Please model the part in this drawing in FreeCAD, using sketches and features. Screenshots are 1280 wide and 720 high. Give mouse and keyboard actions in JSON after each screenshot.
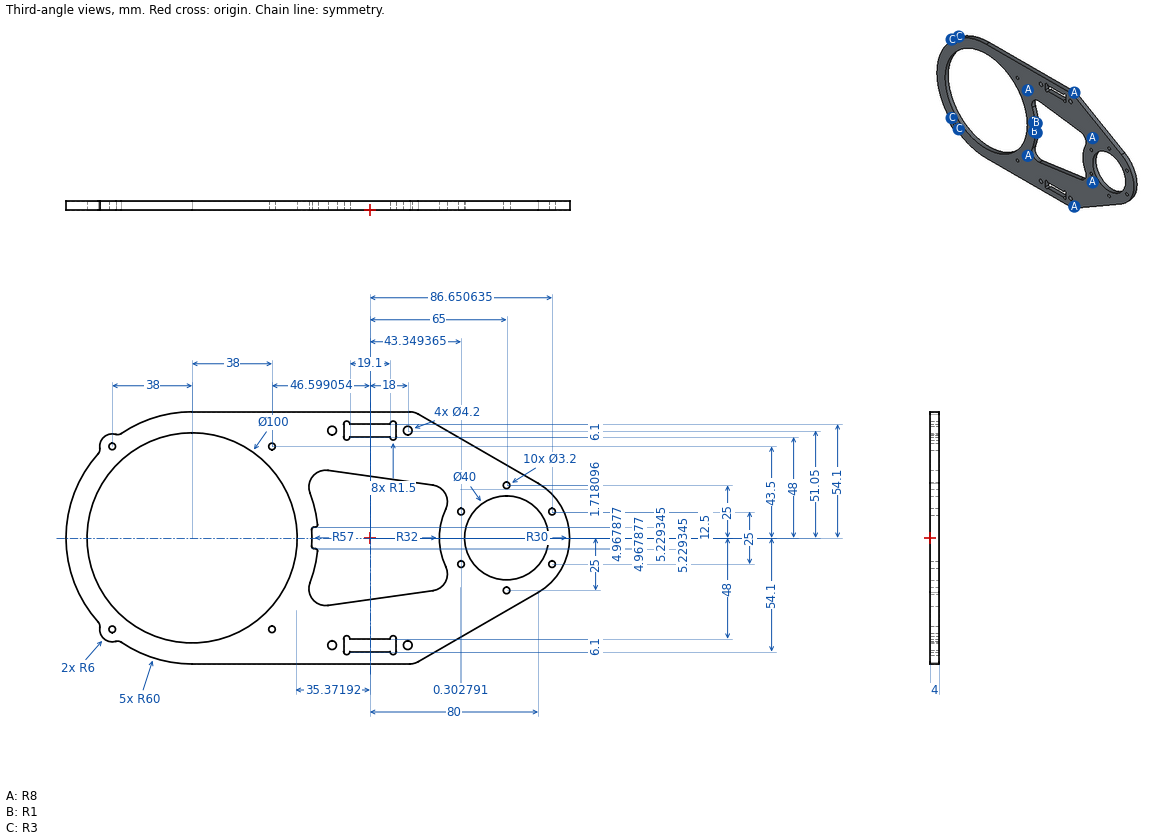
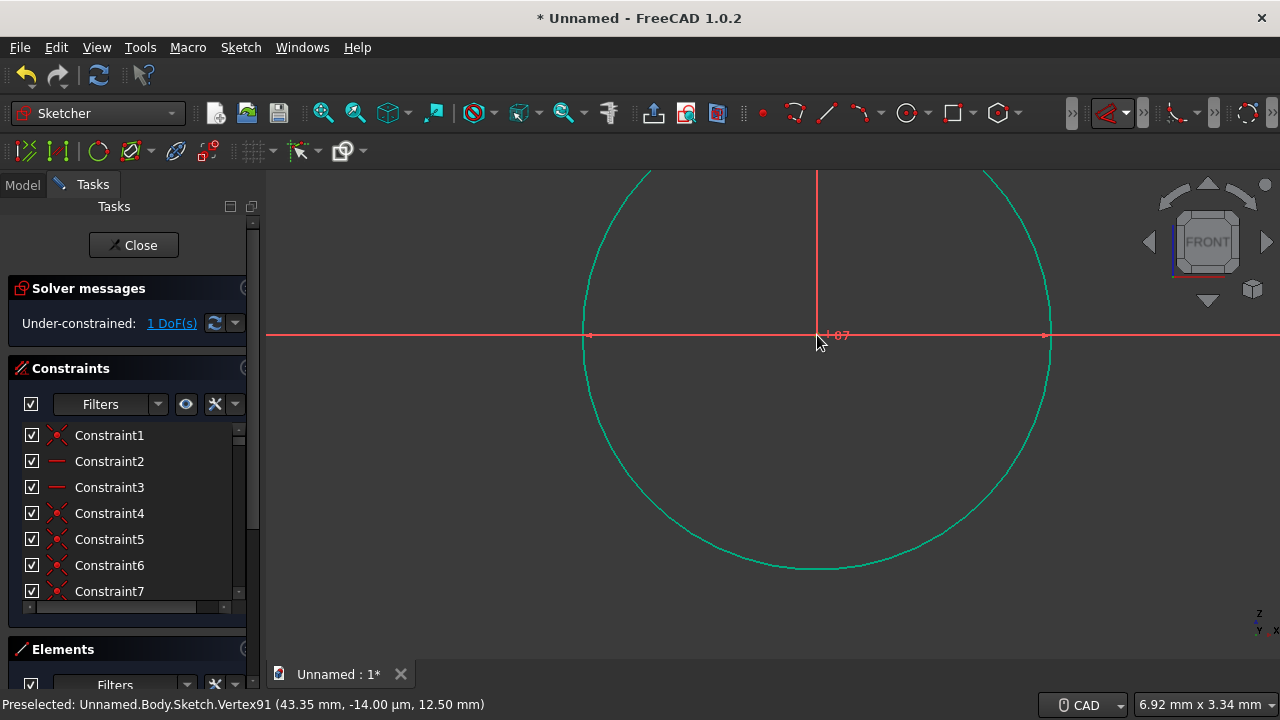
{"action": "left_click", "coordinate": [1128, 114]}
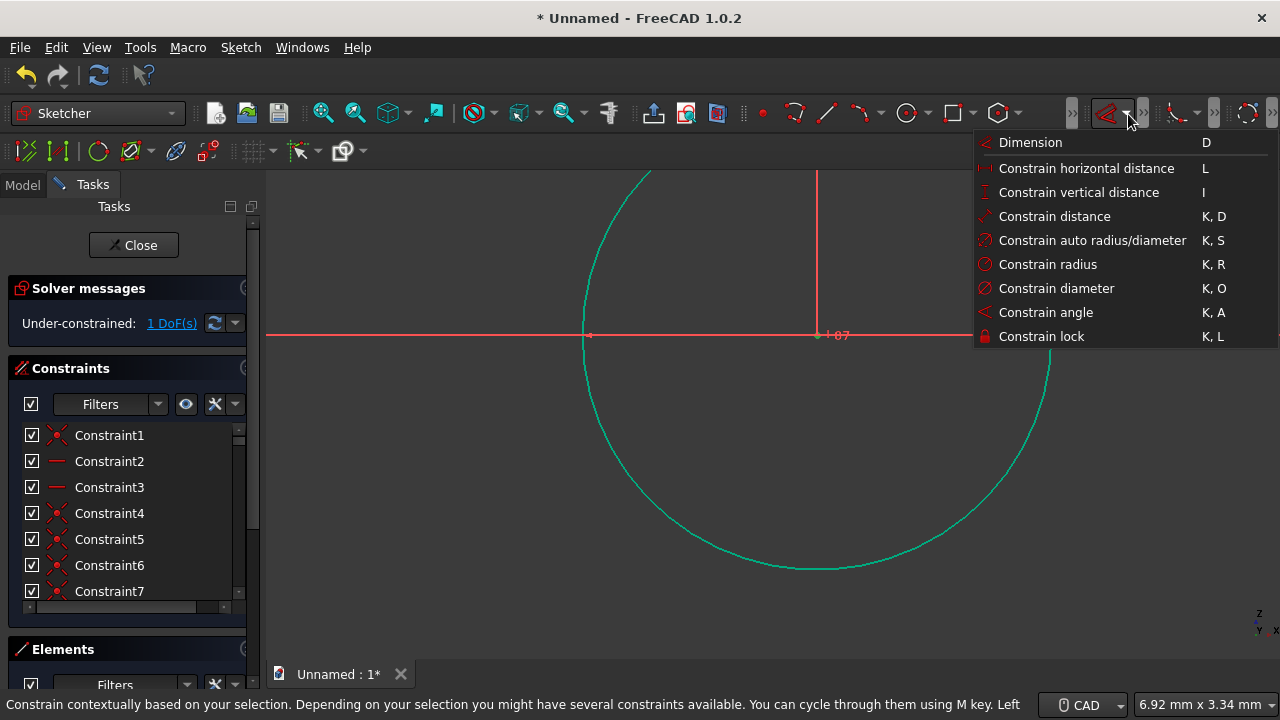
{"action": "left_click", "coordinate": [1126, 168]}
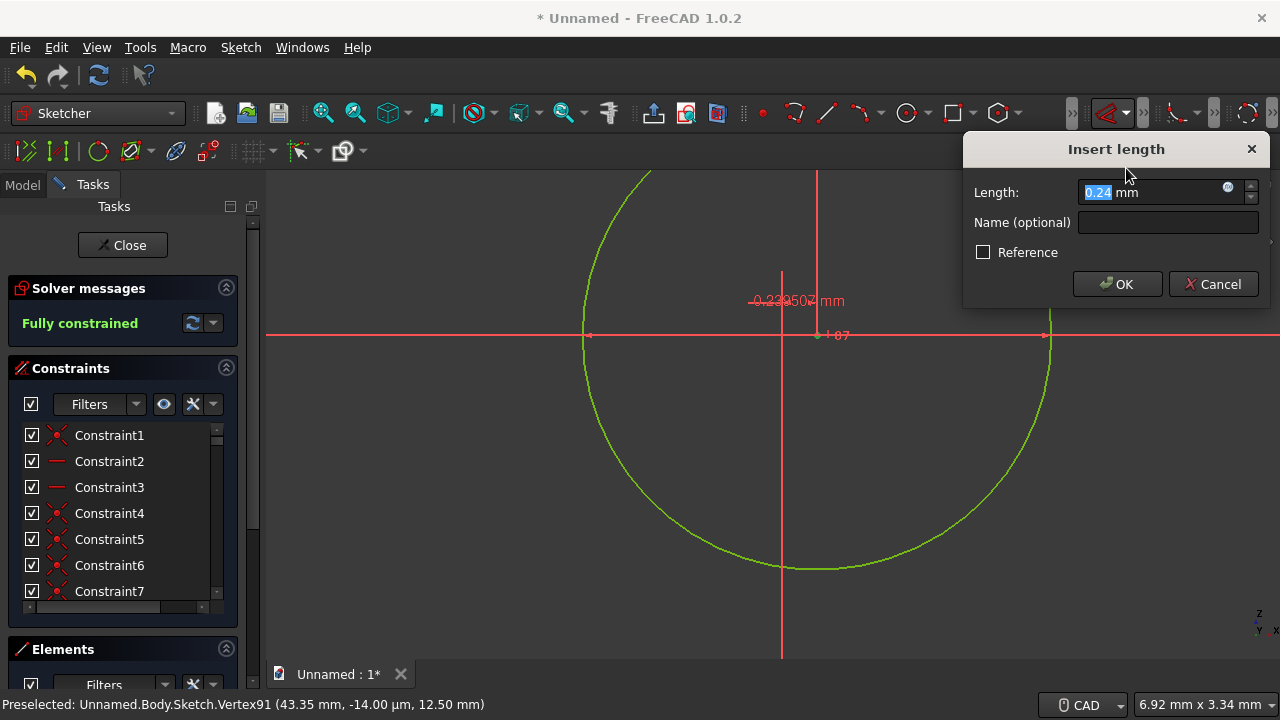
{"action": "type", "text": "0.302791"}
{"action": "key", "text": "Return"}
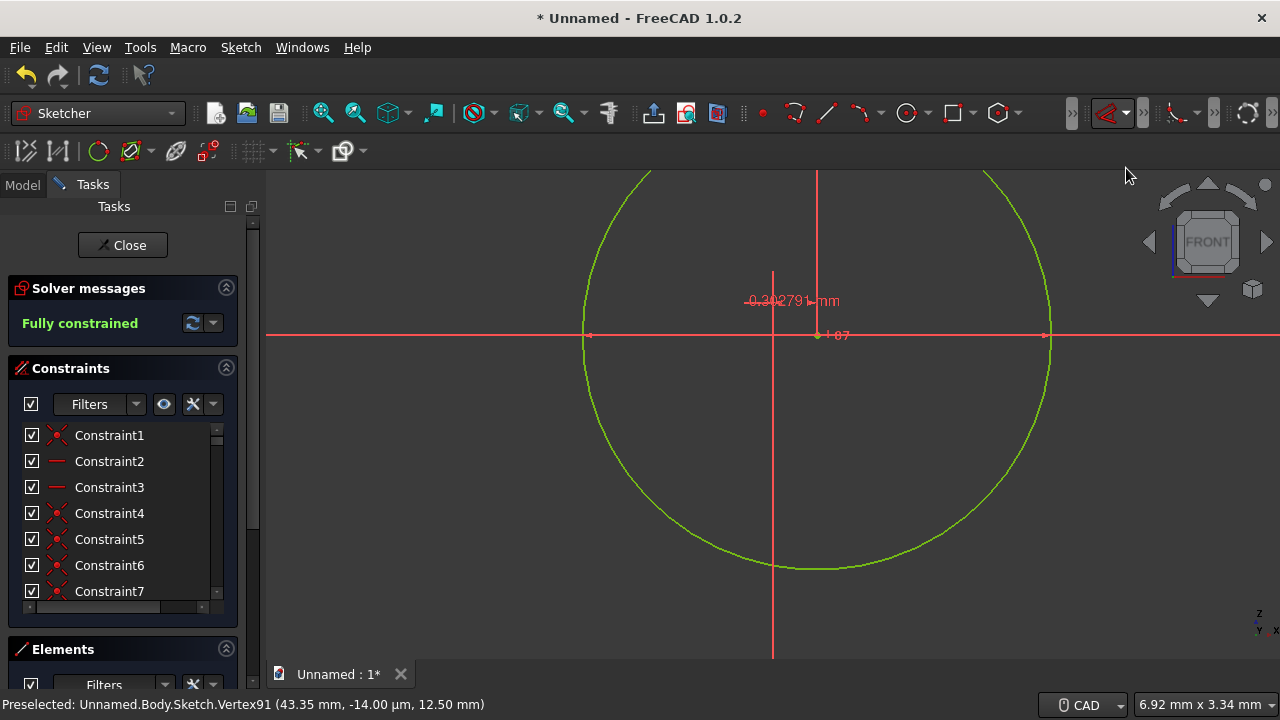
{"action": "left_click", "coordinate": [123, 245]}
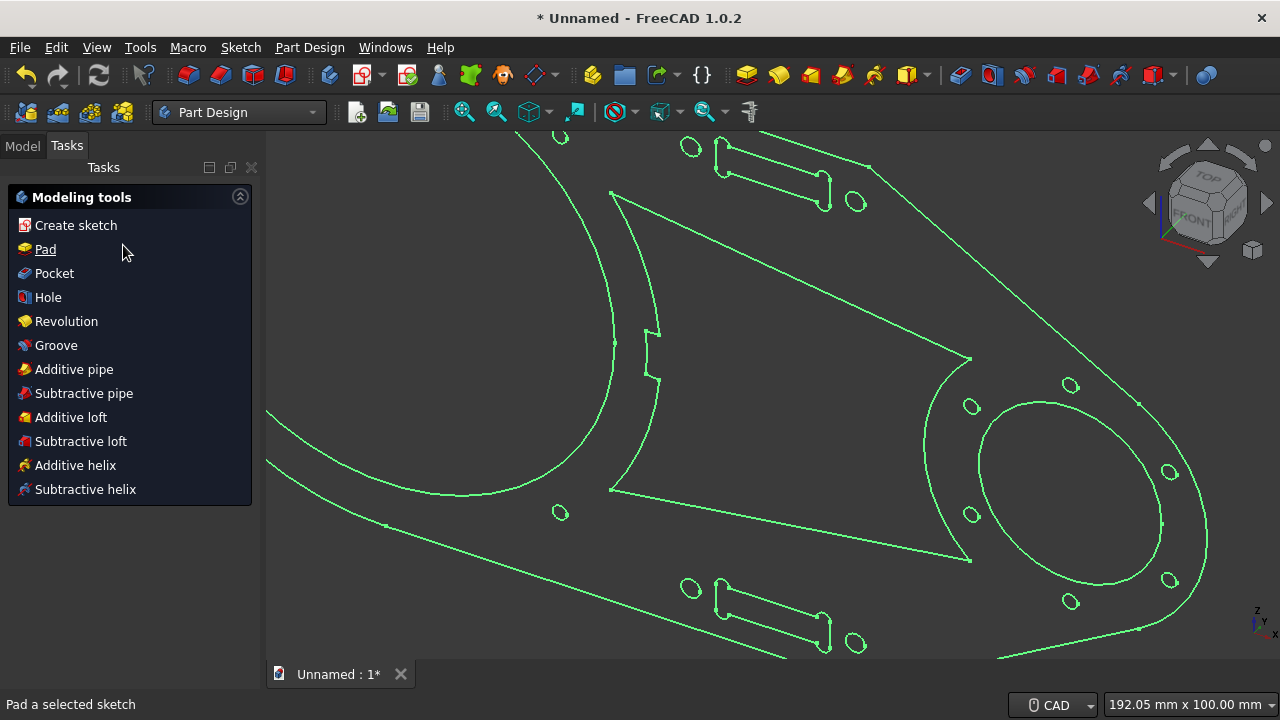
{"action": "left_click", "coordinate": [748, 76]}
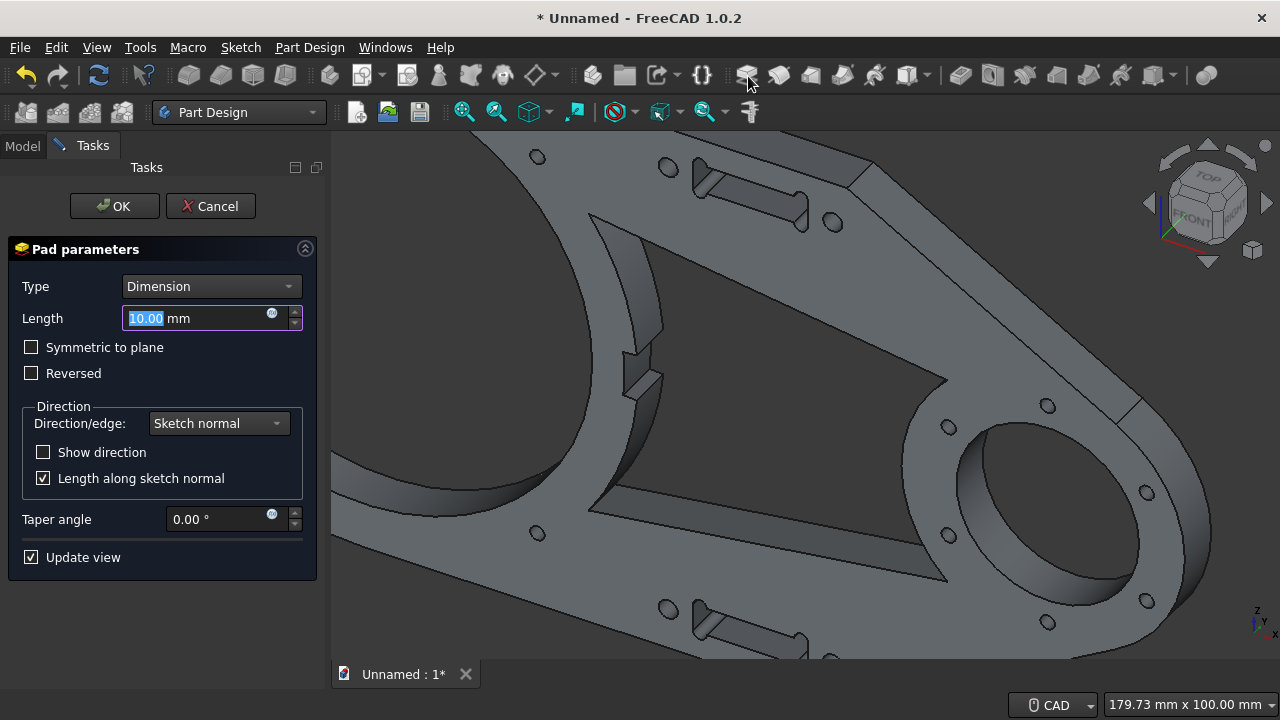
{"action": "type", "text": "4"}
{"action": "key", "text": "Tab"}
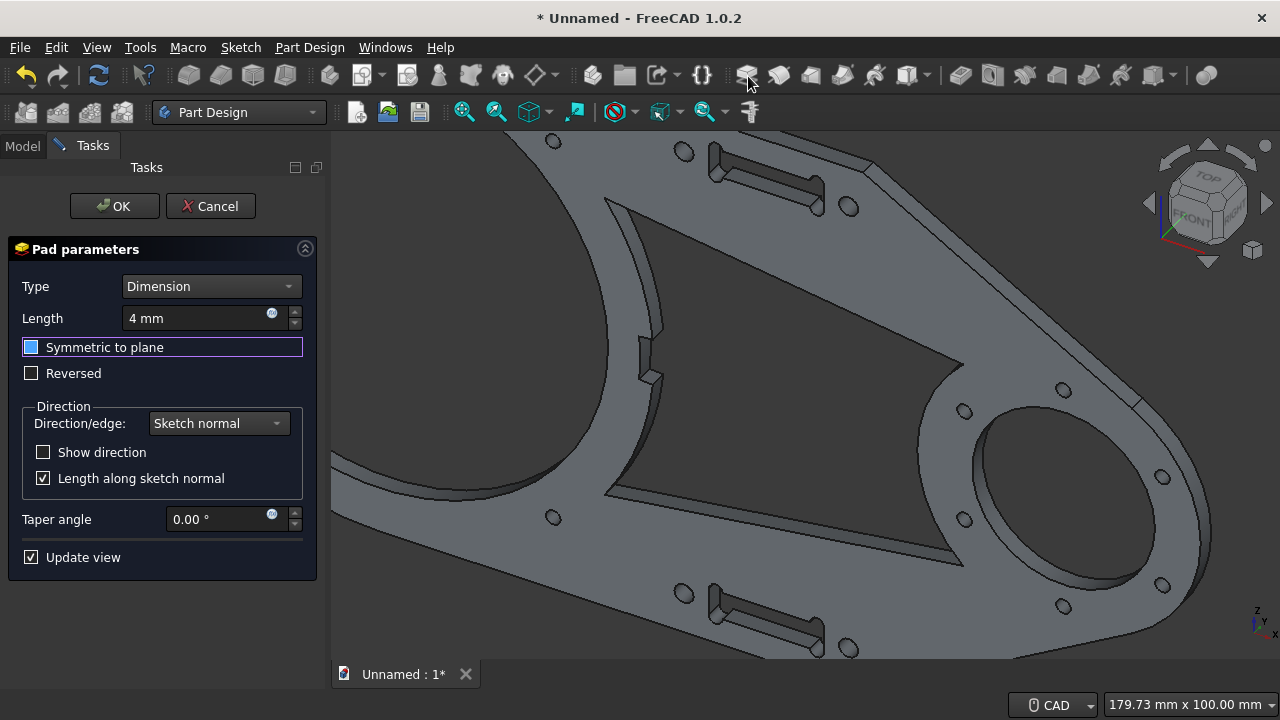
{"action": "left_click", "coordinate": [30, 373]}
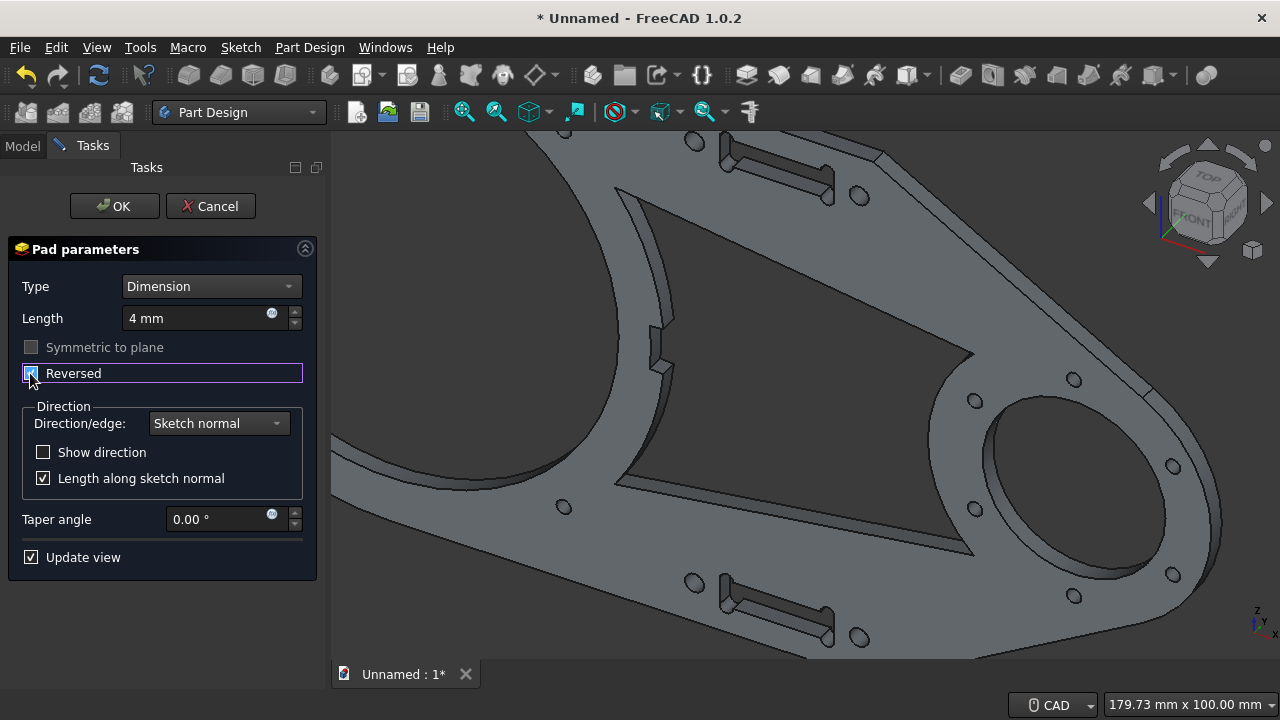
{"action": "left_click", "coordinate": [115, 206]}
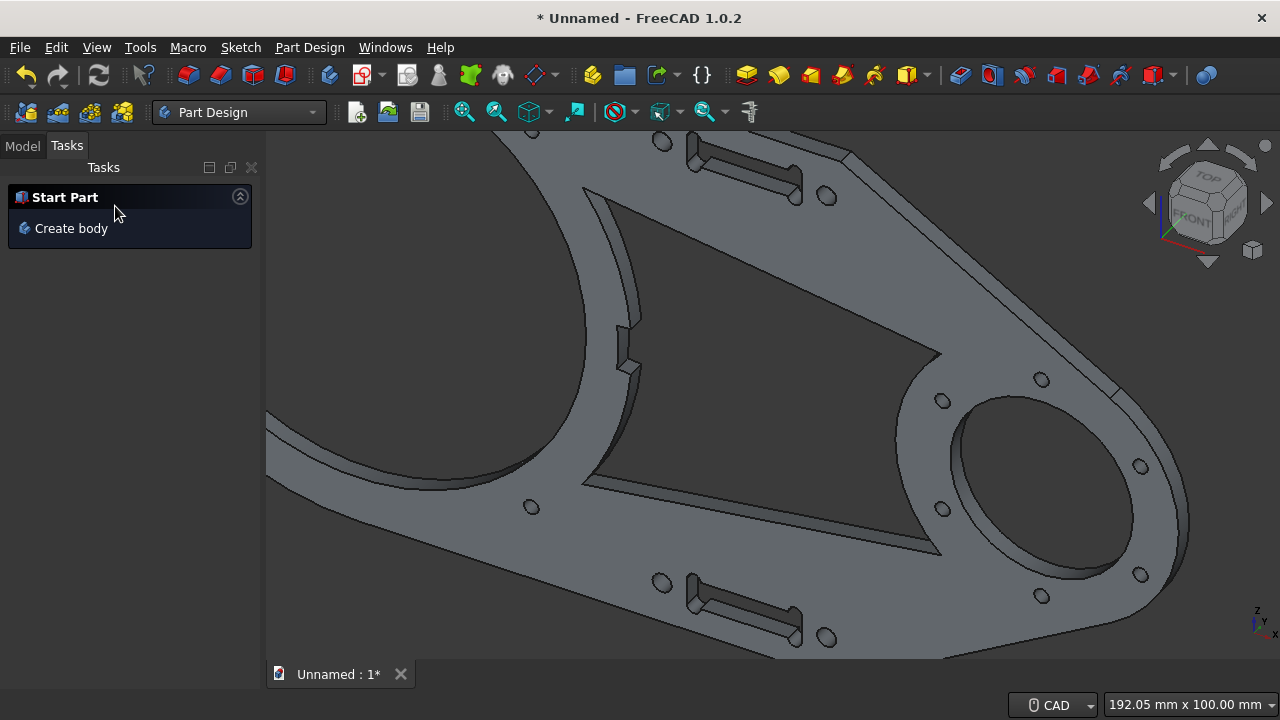
{"action": "left_click", "coordinate": [466, 112]}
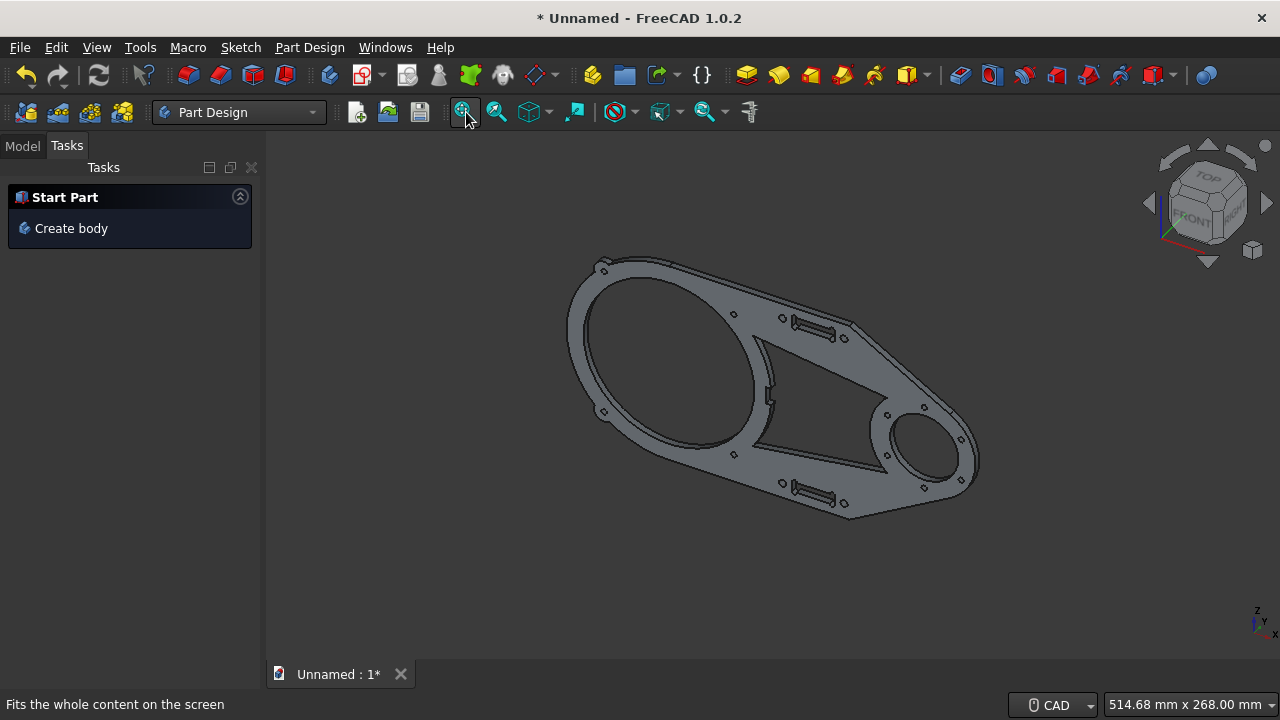
{"action": "scroll", "coordinate": [755, 443], "scroll_direction": "up", "scroll_amount": 9}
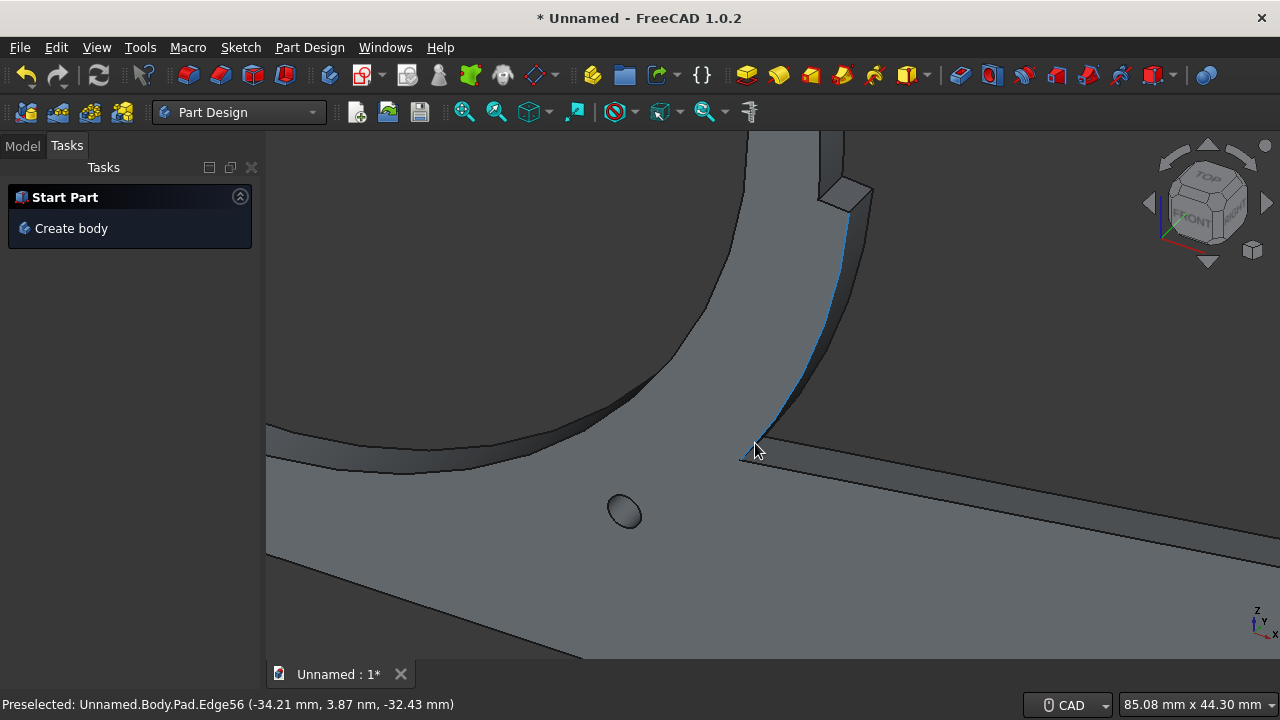
{"action": "key", "text": "v f"}